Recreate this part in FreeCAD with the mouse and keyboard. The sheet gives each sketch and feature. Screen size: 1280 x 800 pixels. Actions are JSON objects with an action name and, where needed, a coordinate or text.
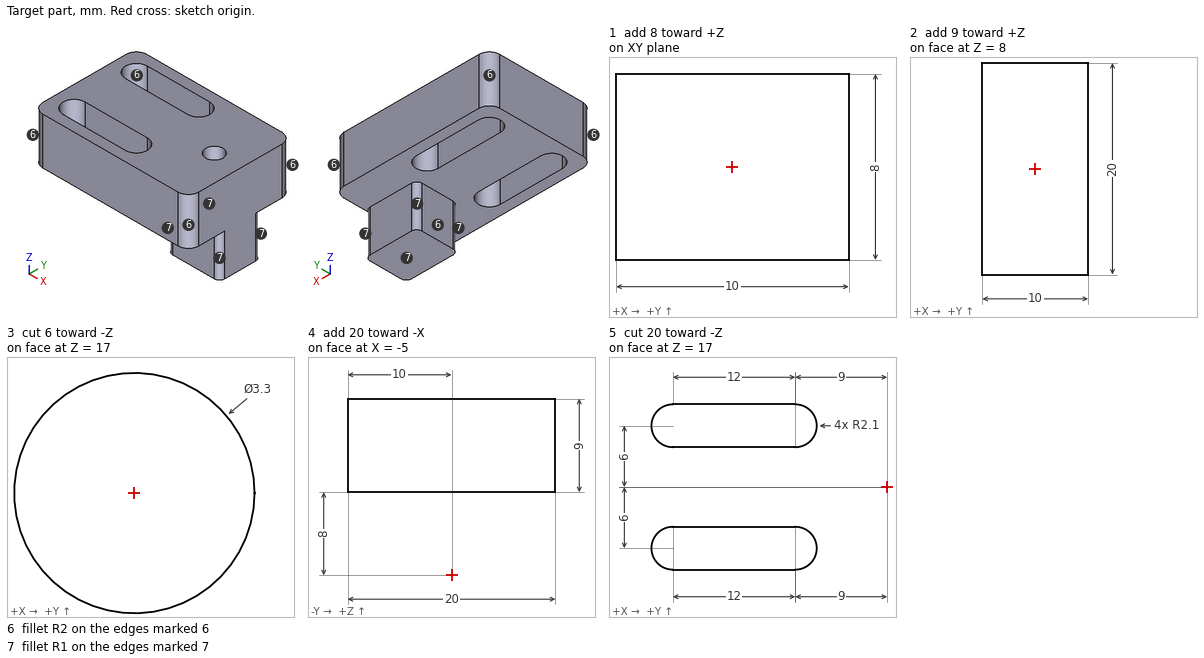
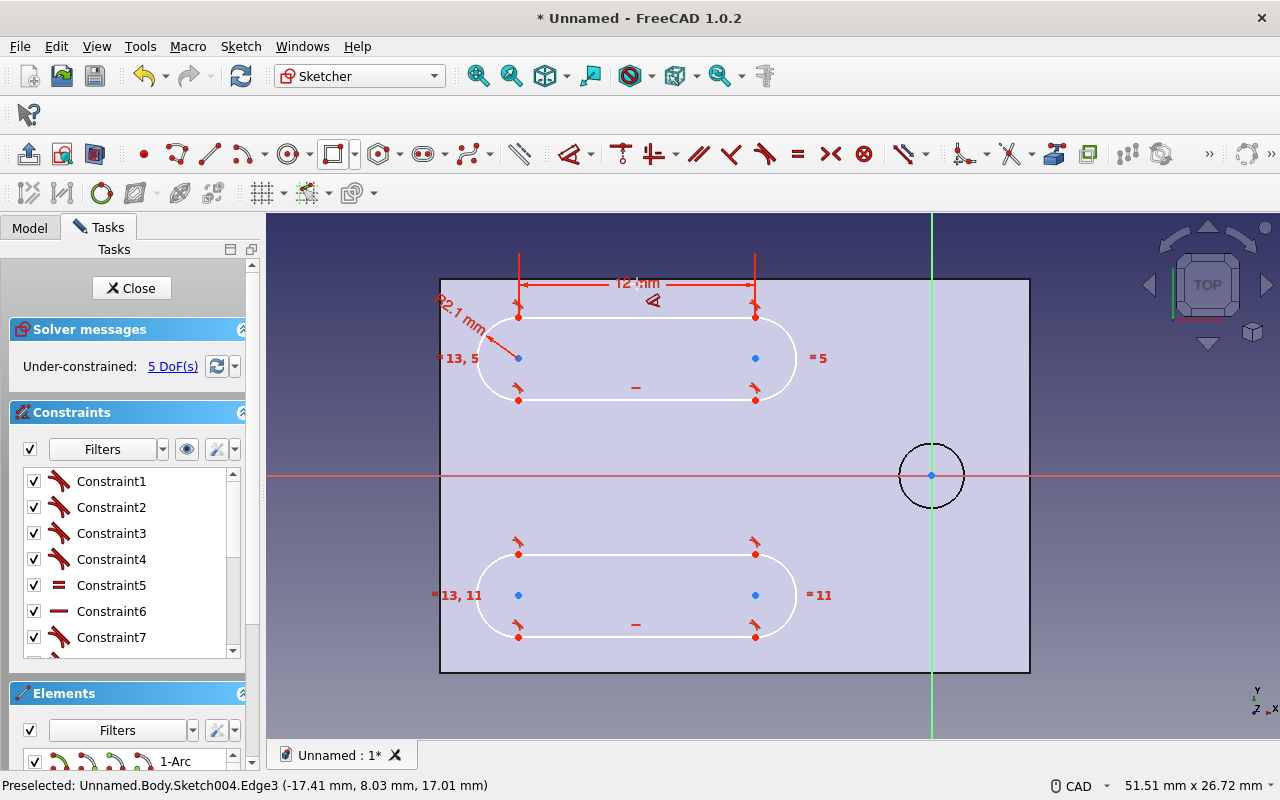
{"action": "left_click", "coordinate": [589, 555]}
{"action": "left_click", "coordinate": [637, 589]}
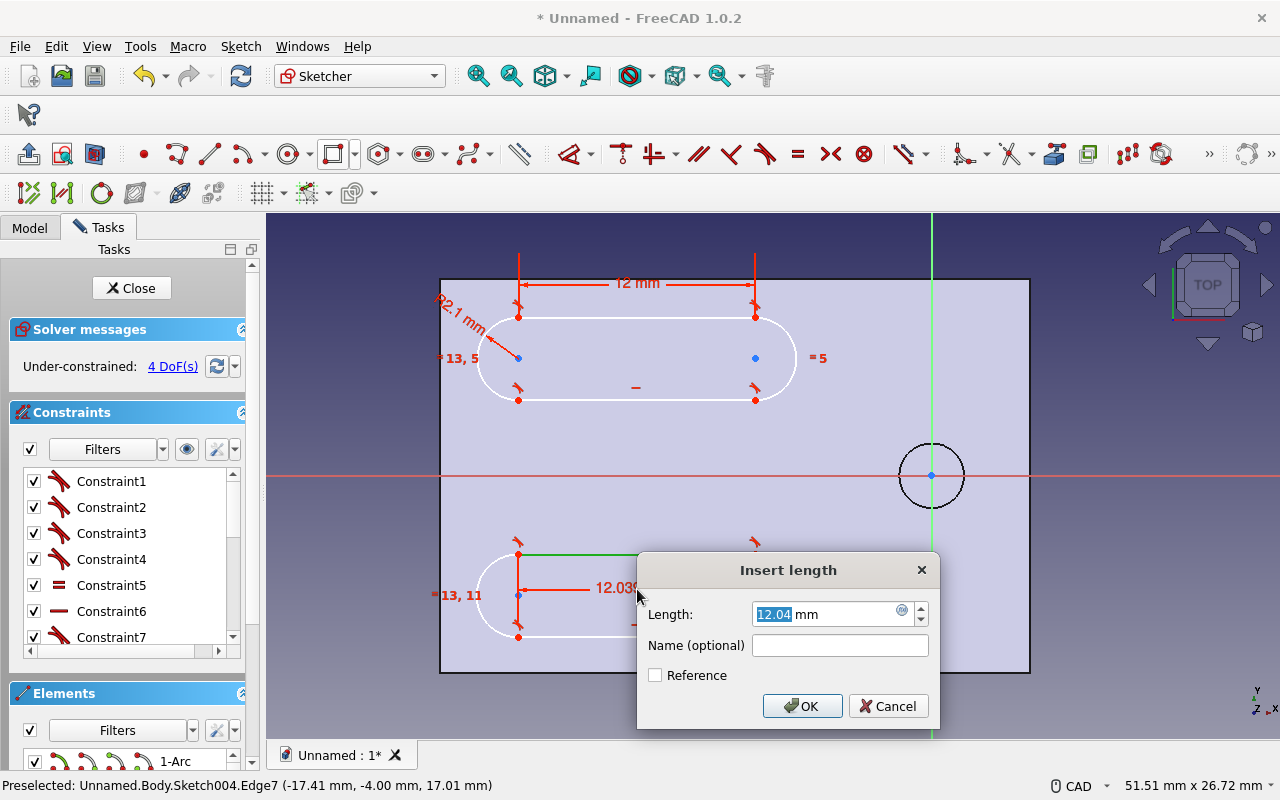
{"action": "type", "text": "12"}
{"action": "key", "text": "Return"}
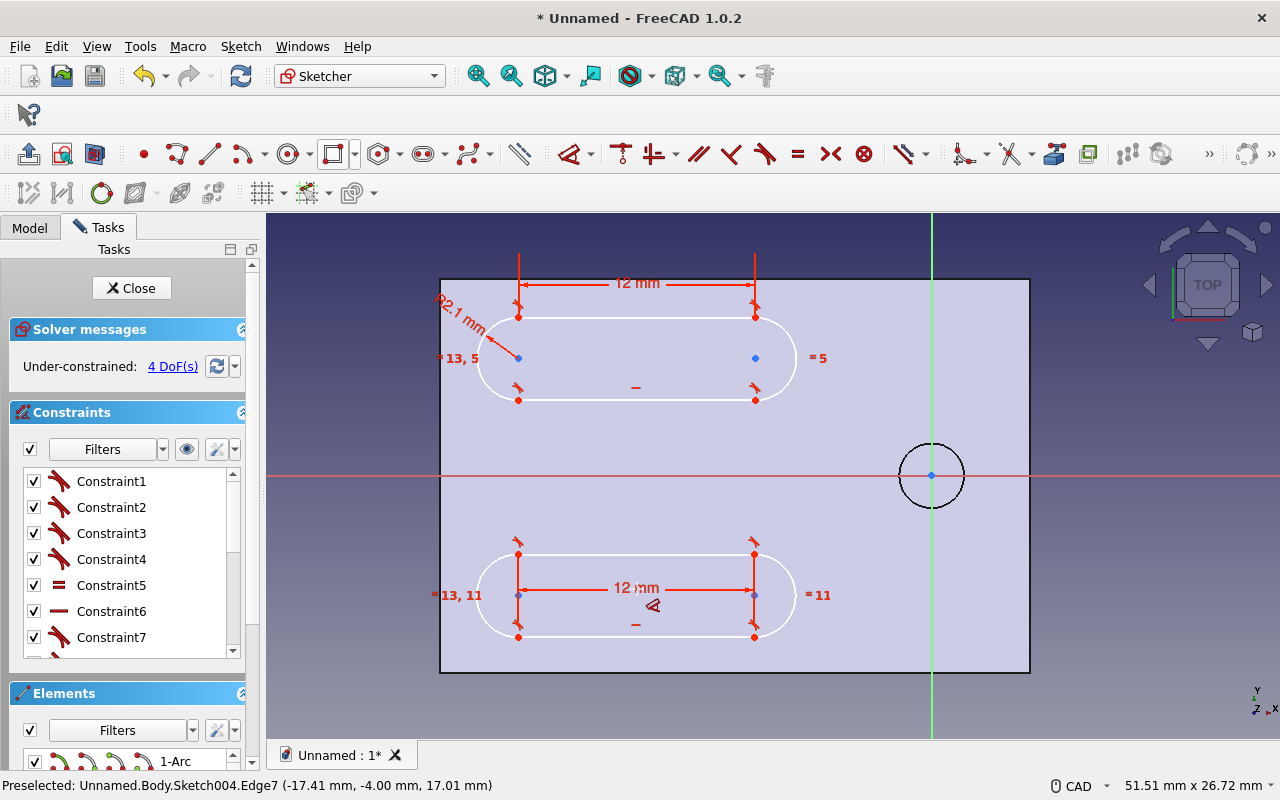
{"action": "left_click", "coordinate": [755, 400]}
{"action": "left_click", "coordinate": [843, 366]}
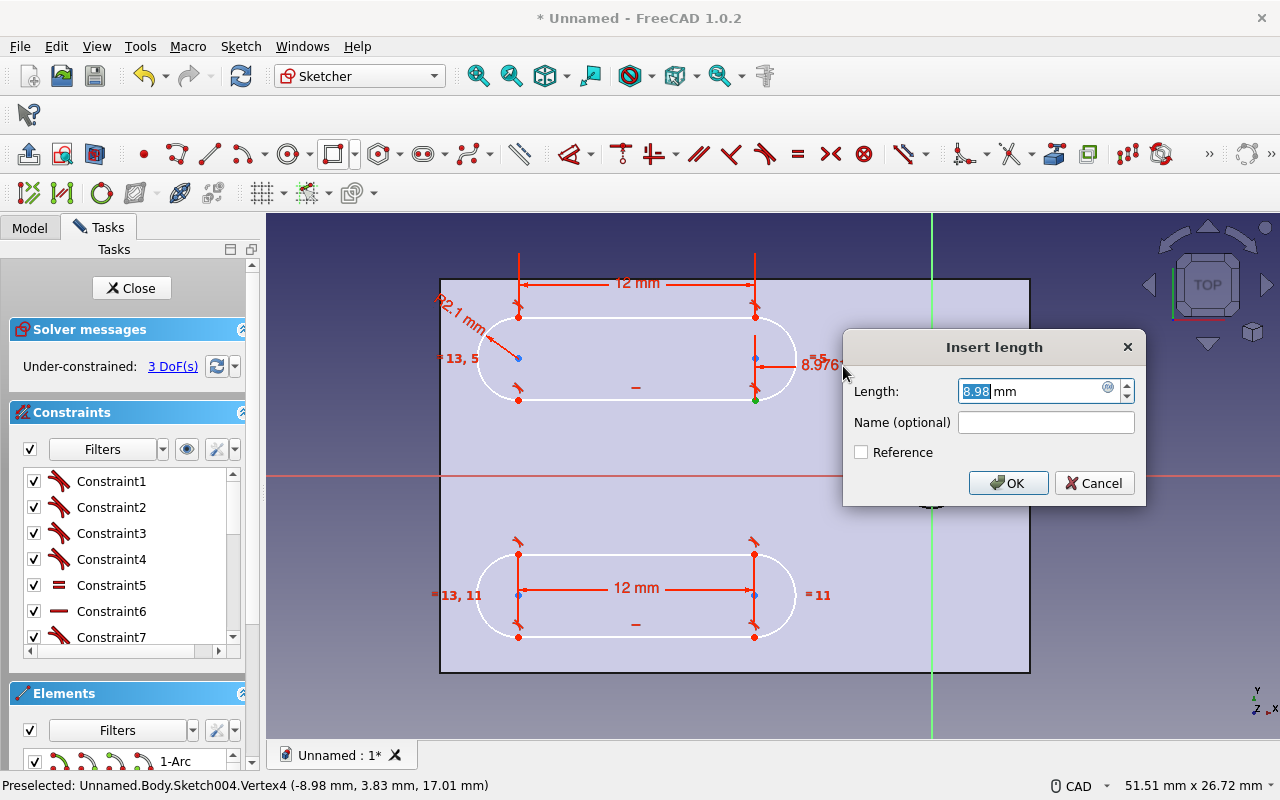
{"action": "type", "text": "9"}
{"action": "key", "text": "Return"}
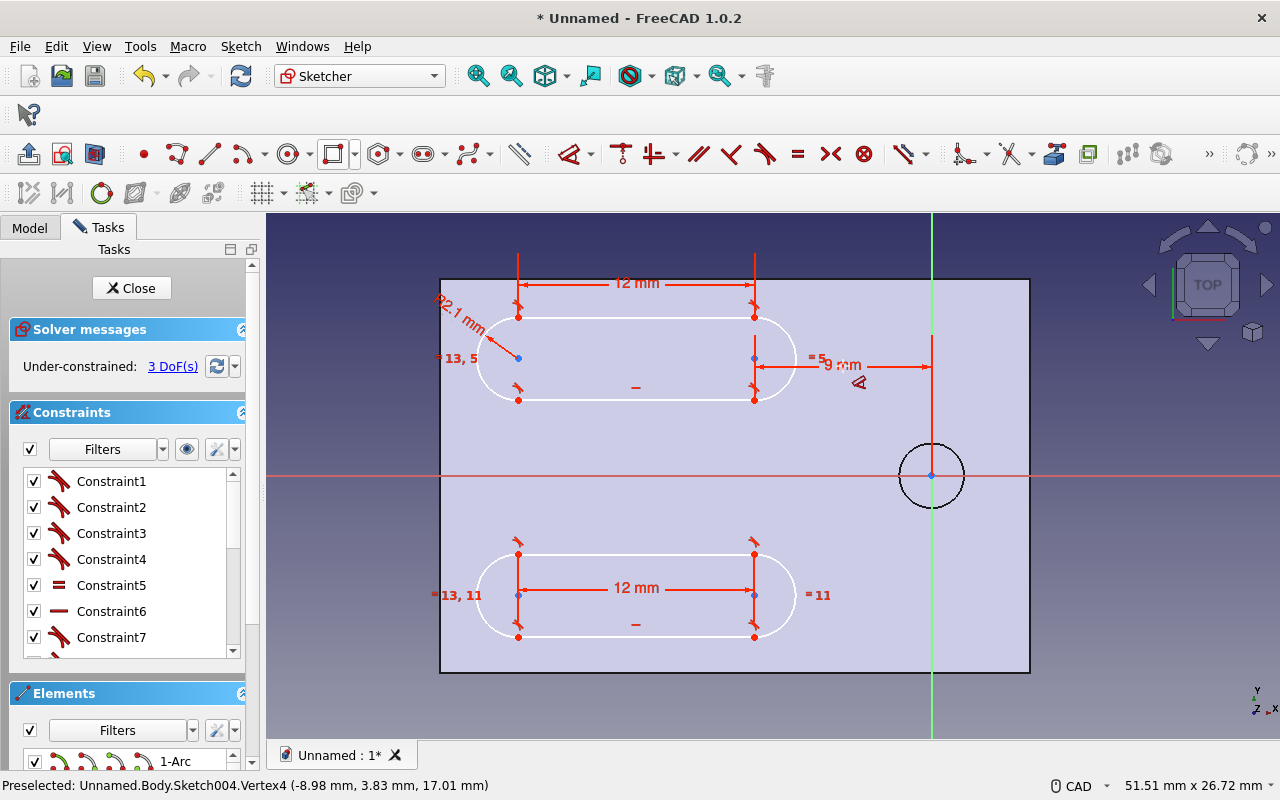
{"action": "left_click", "coordinate": [754, 637]}
{"action": "left_click", "coordinate": [843, 671]}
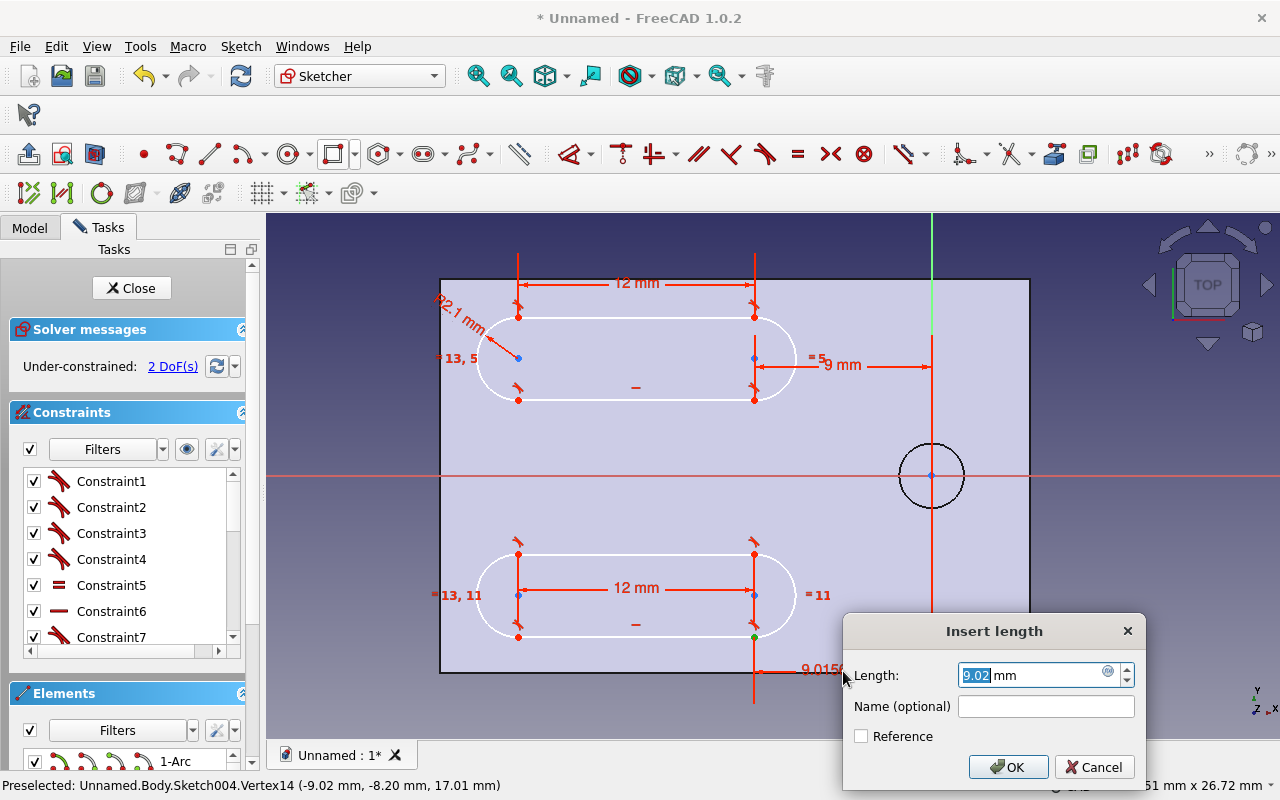
{"action": "type", "text": "9"}
{"action": "key", "text": "Return"}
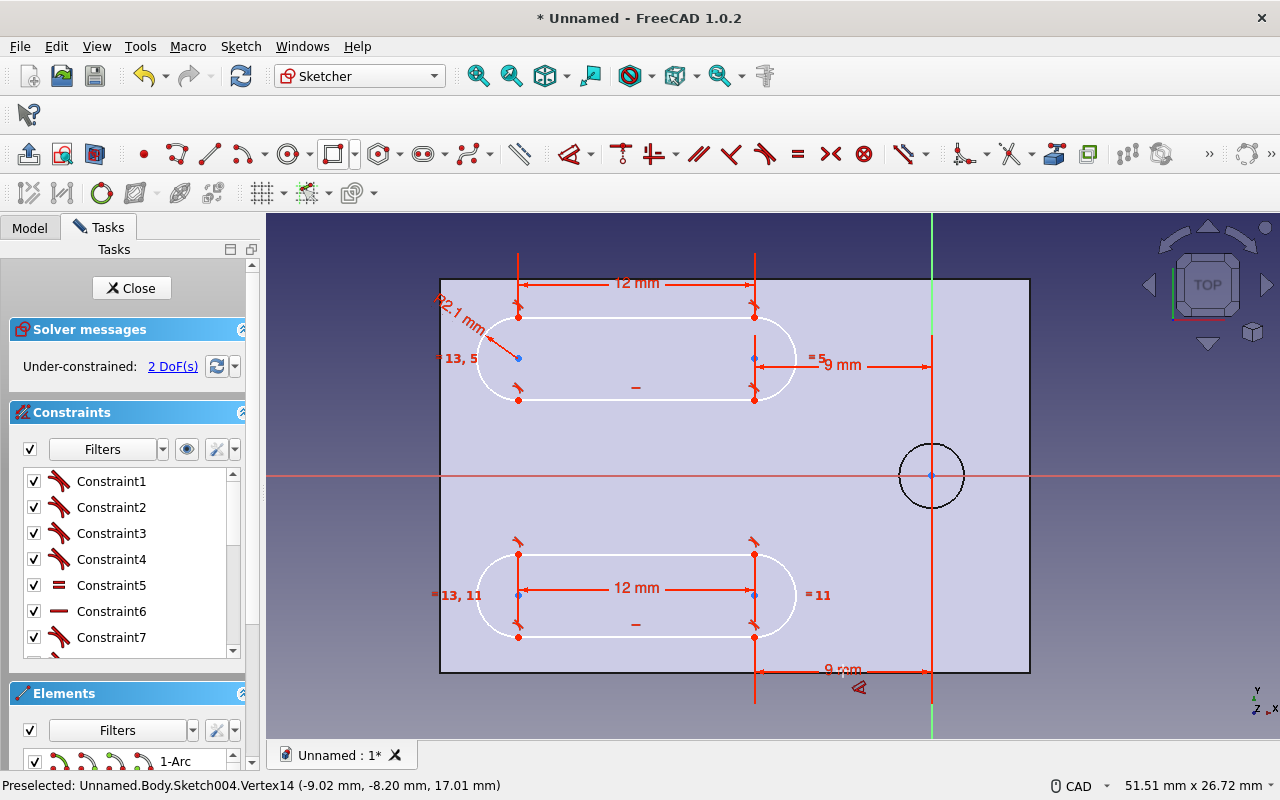
{"action": "left_click", "coordinate": [518, 359]}
{"action": "left_click", "coordinate": [966, 417]}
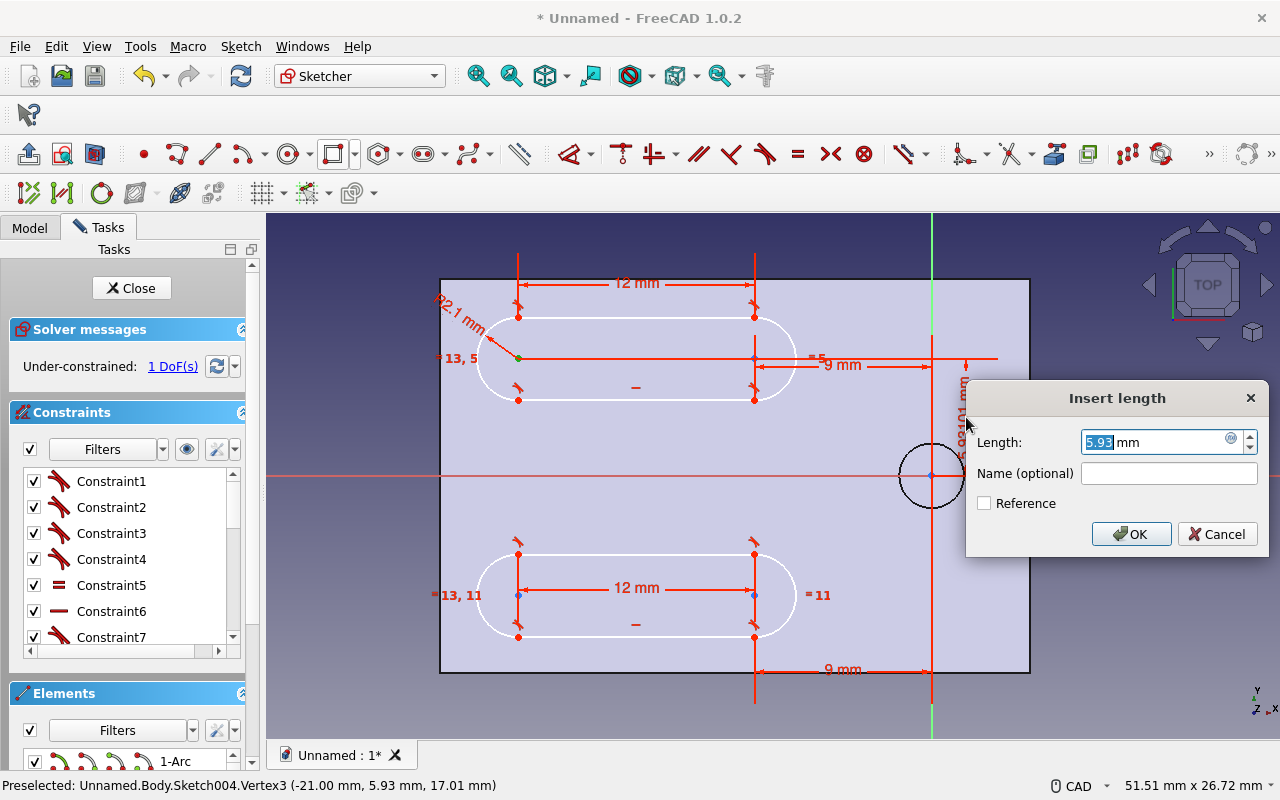
{"action": "type", "text": "6"}
{"action": "key", "text": "Return"}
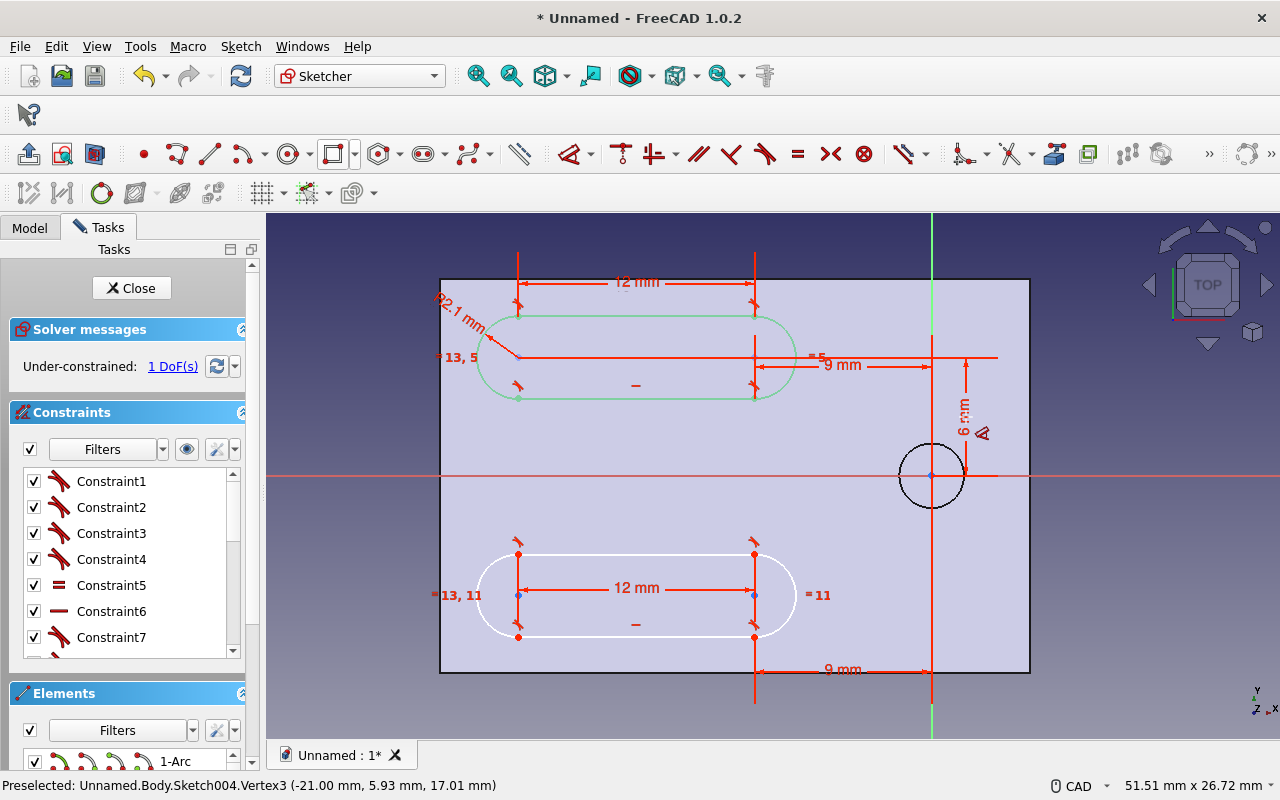
{"action": "left_click", "coordinate": [518, 596]}
{"action": "left_click", "coordinate": [966, 536]}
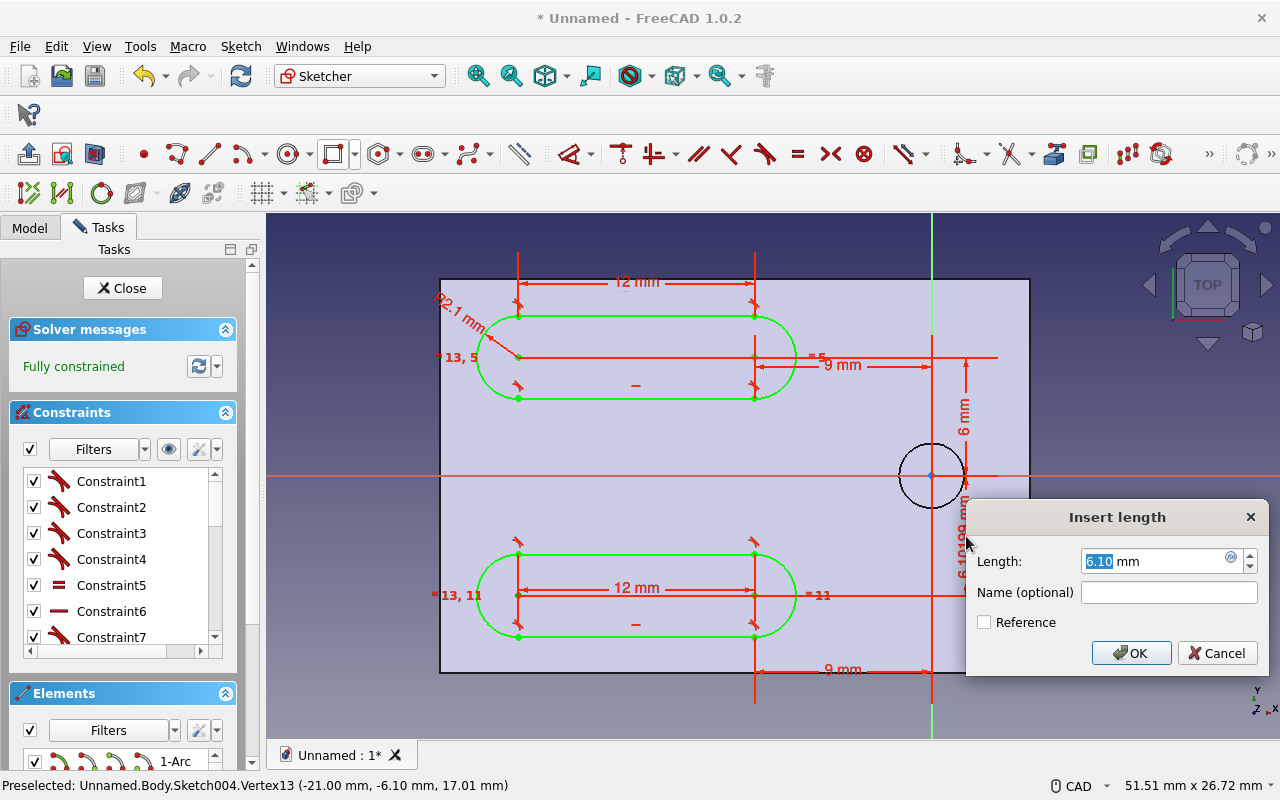
{"action": "type", "text": "6"}
{"action": "key", "text": "Return"}
{"action": "key", "text": "Escape"}